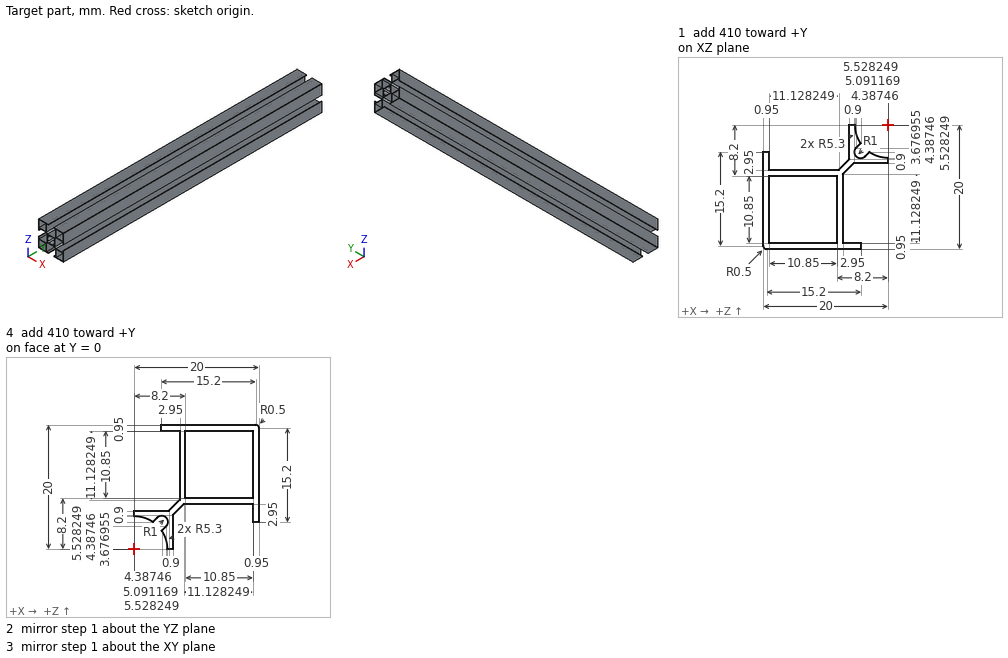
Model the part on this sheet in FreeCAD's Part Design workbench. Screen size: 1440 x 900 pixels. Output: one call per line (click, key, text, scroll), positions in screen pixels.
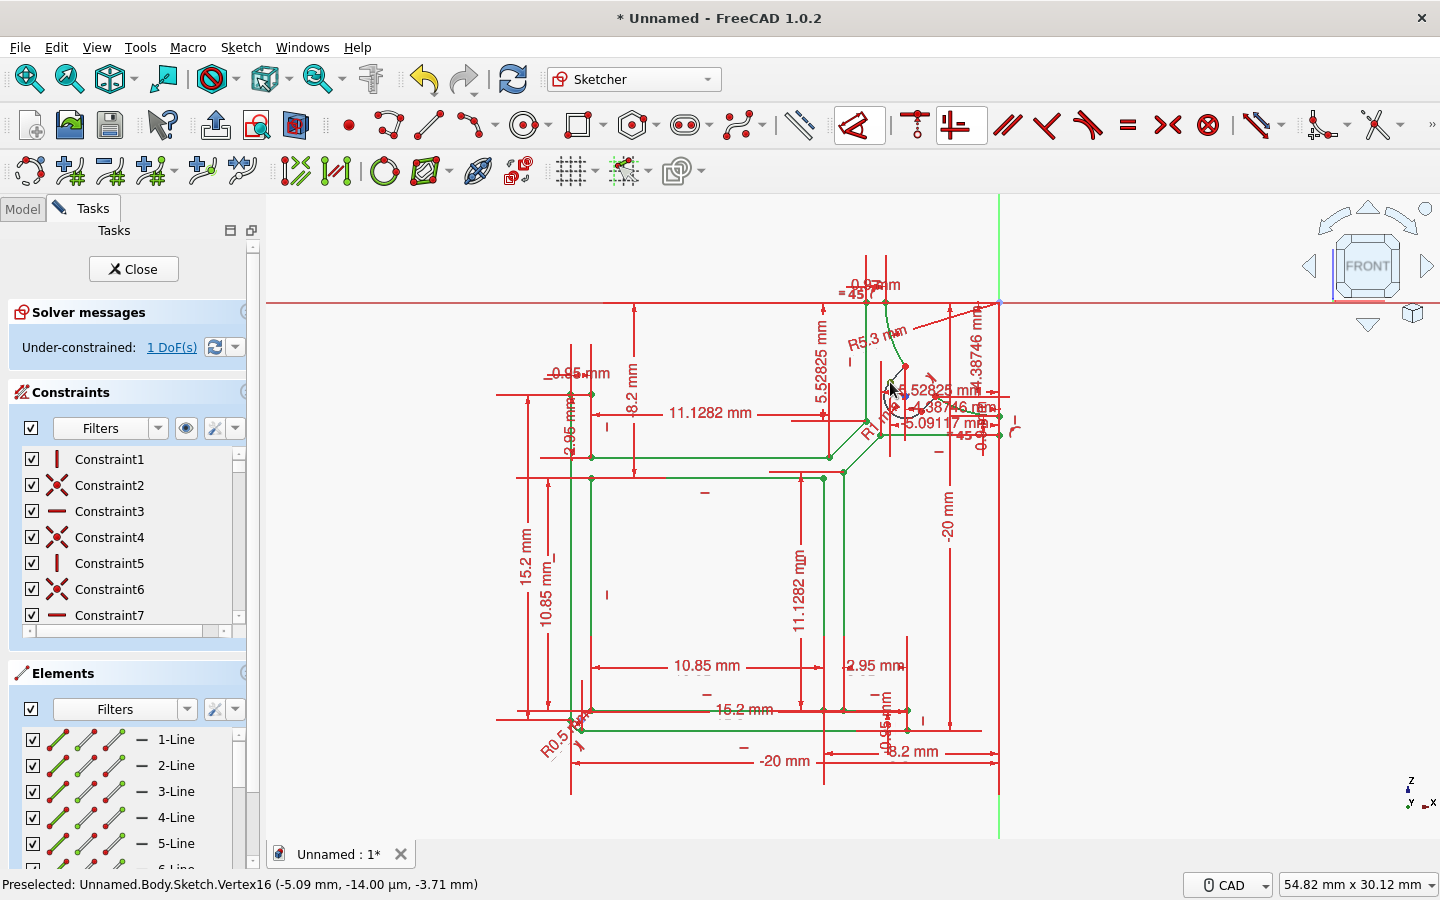
click(880, 126)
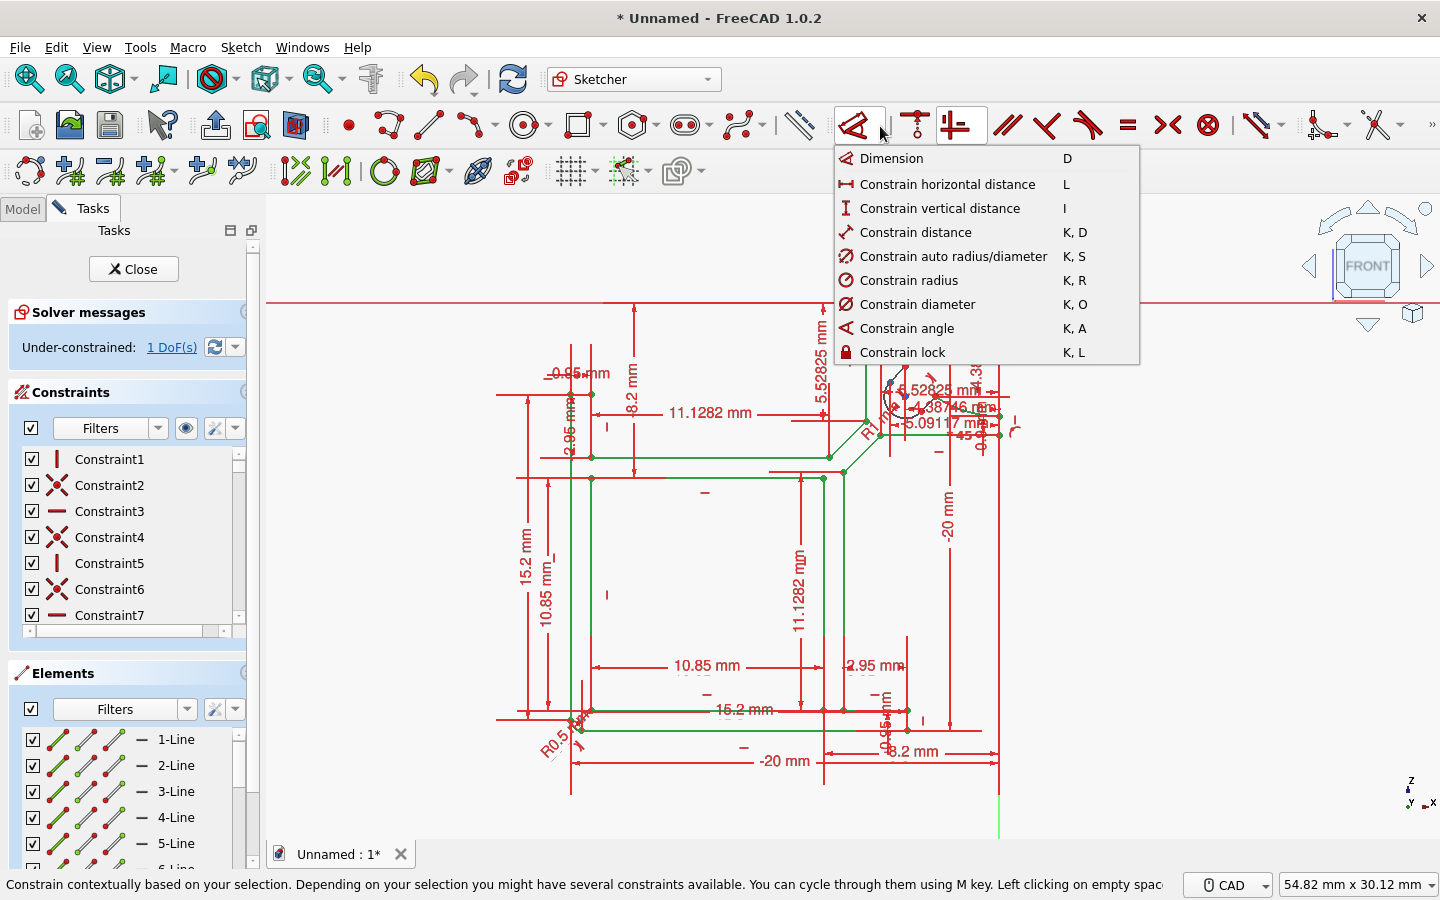
click(987, 208)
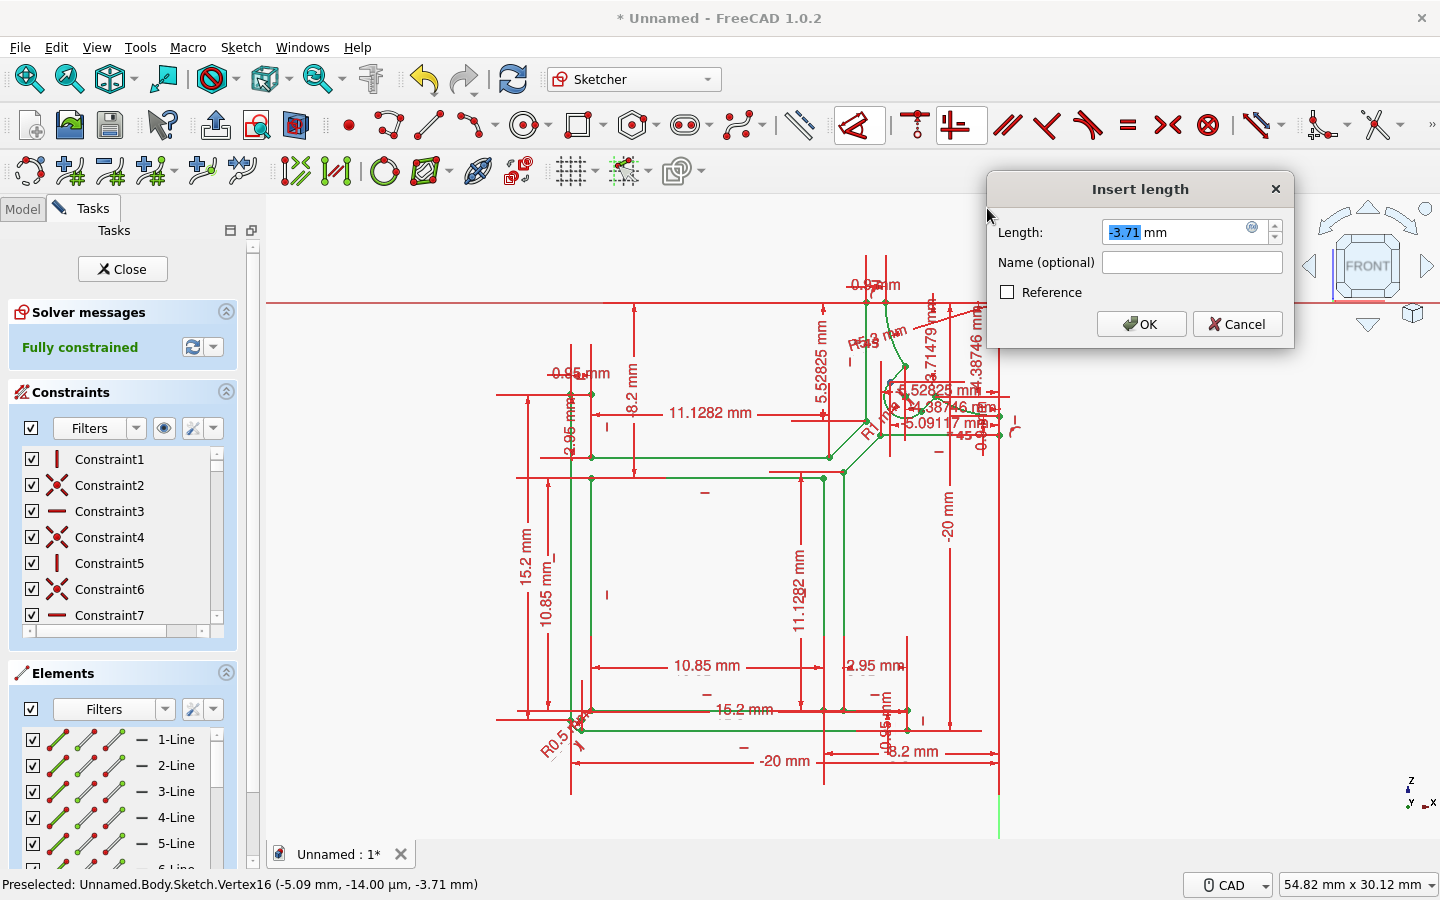
text(-3.676955)
key(Return)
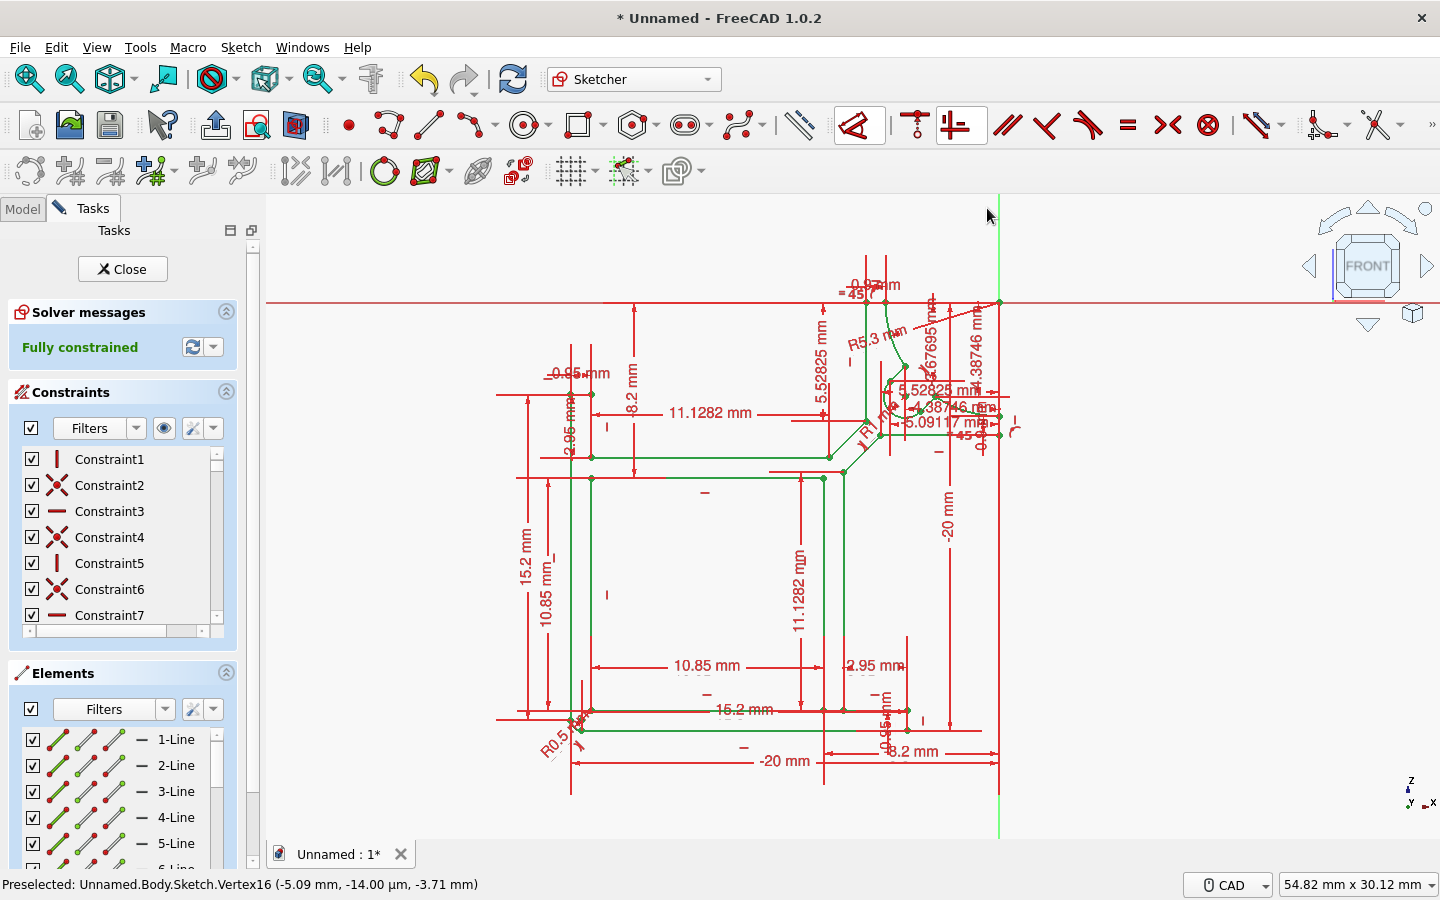
click(123, 269)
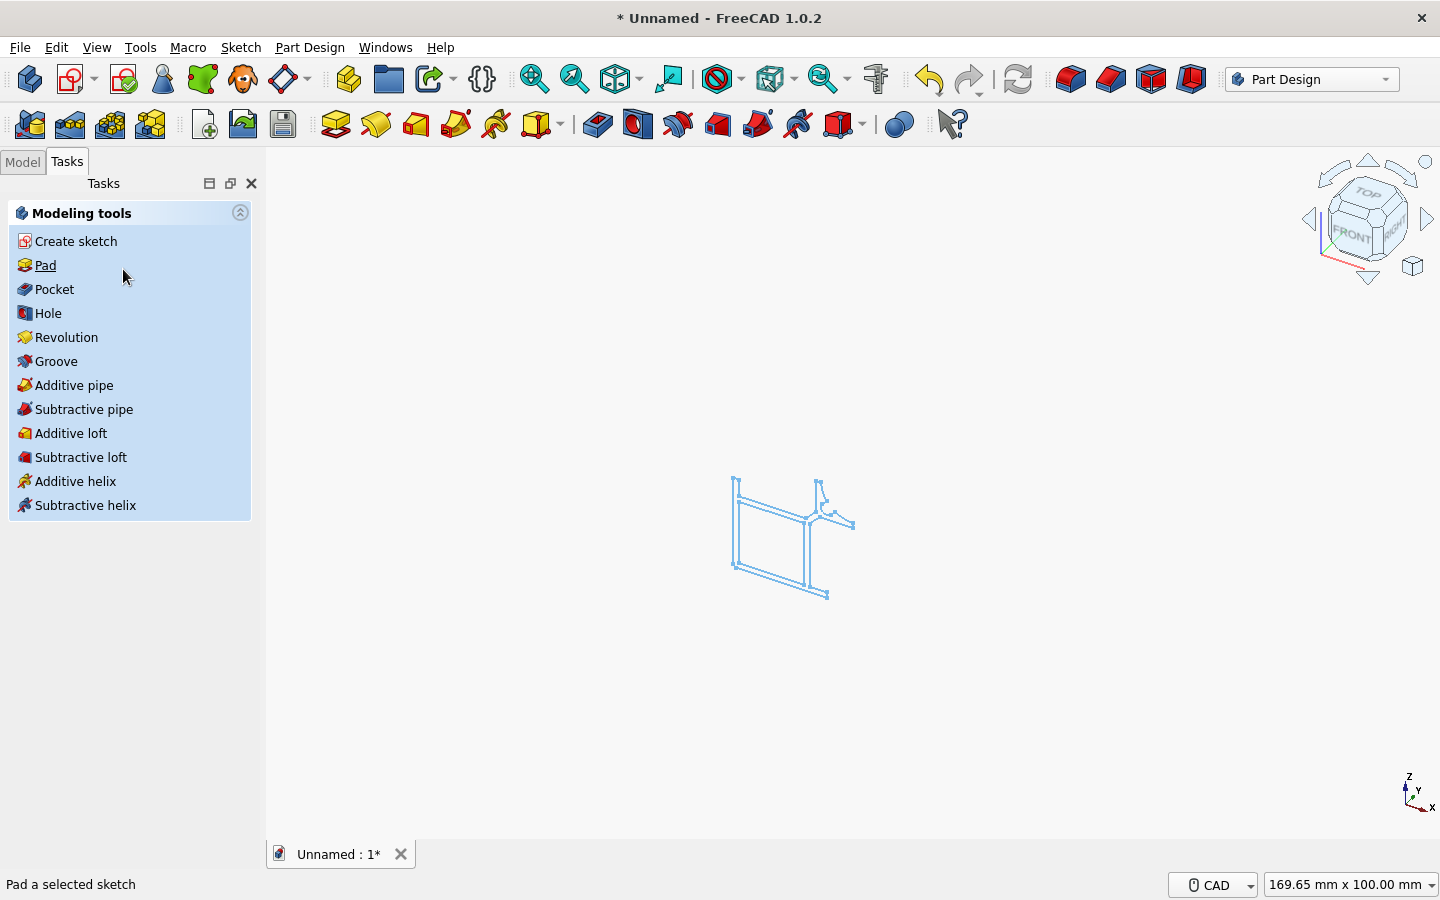
click(336, 124)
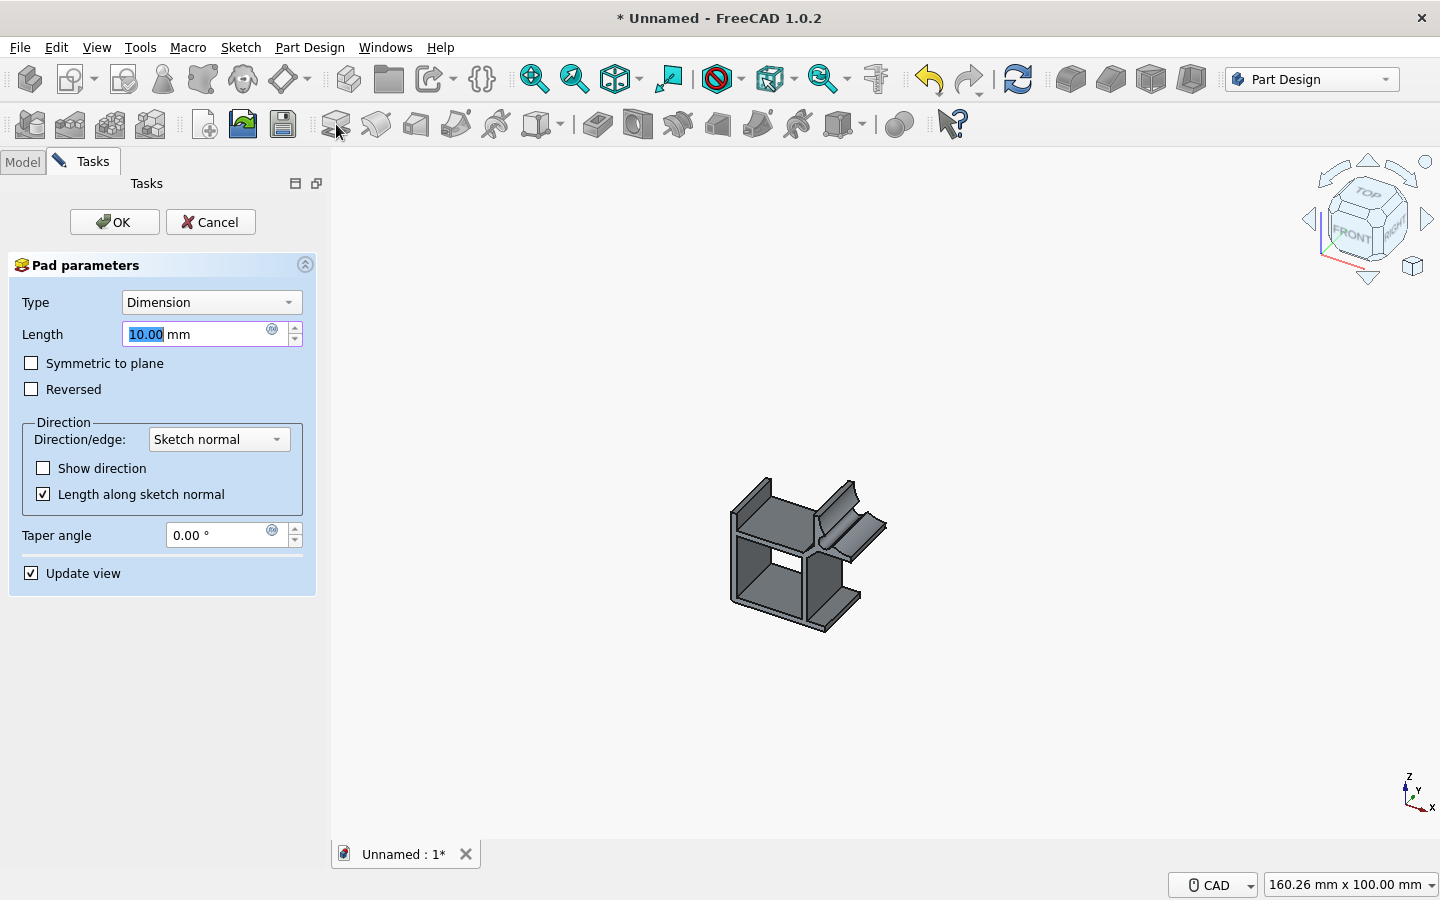
text(410)
key(Tab)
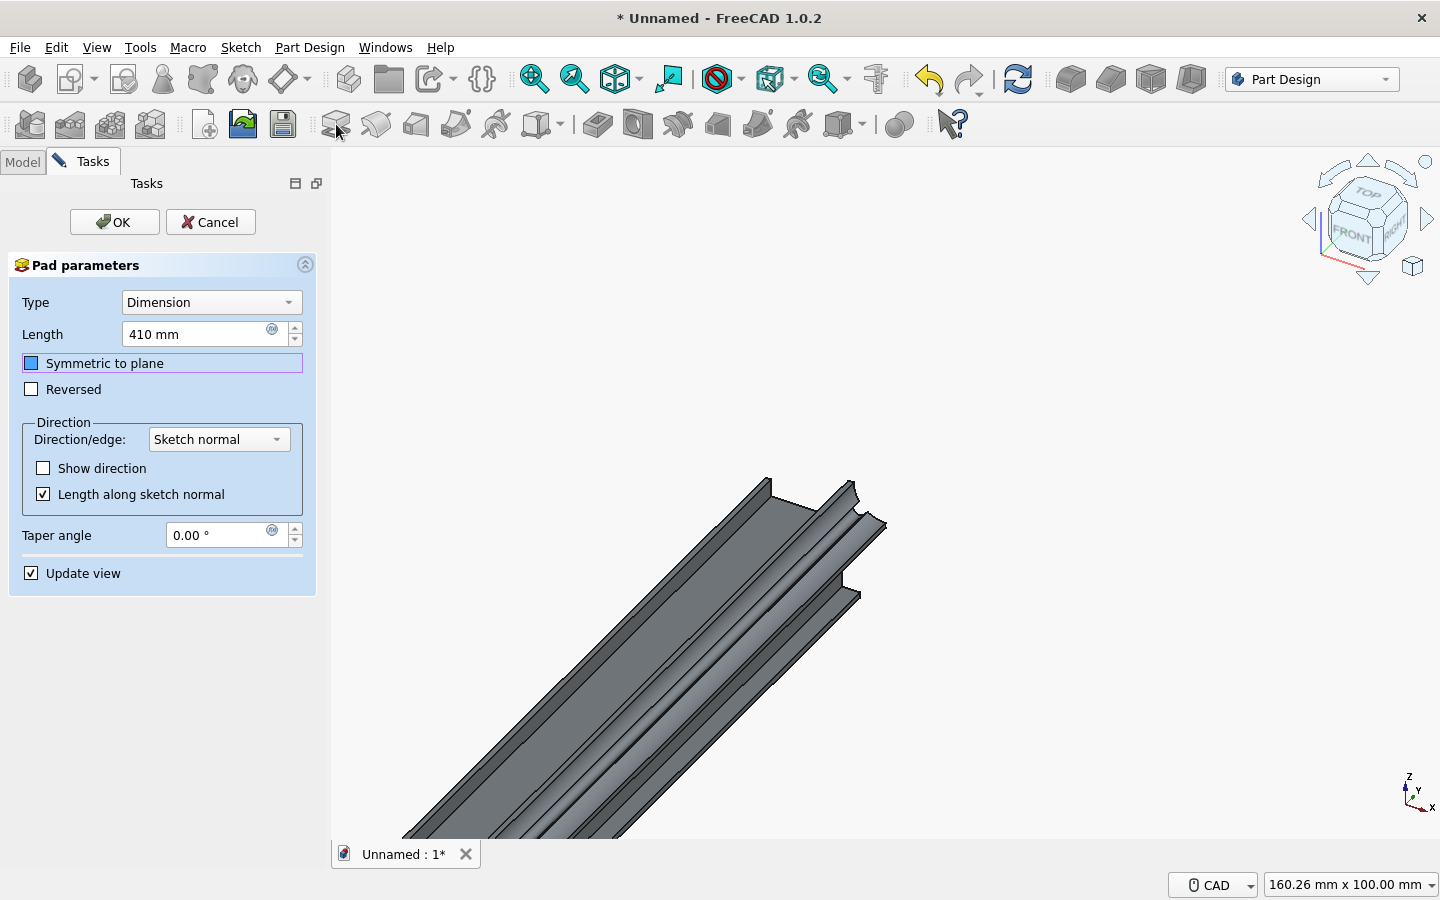
click(30, 389)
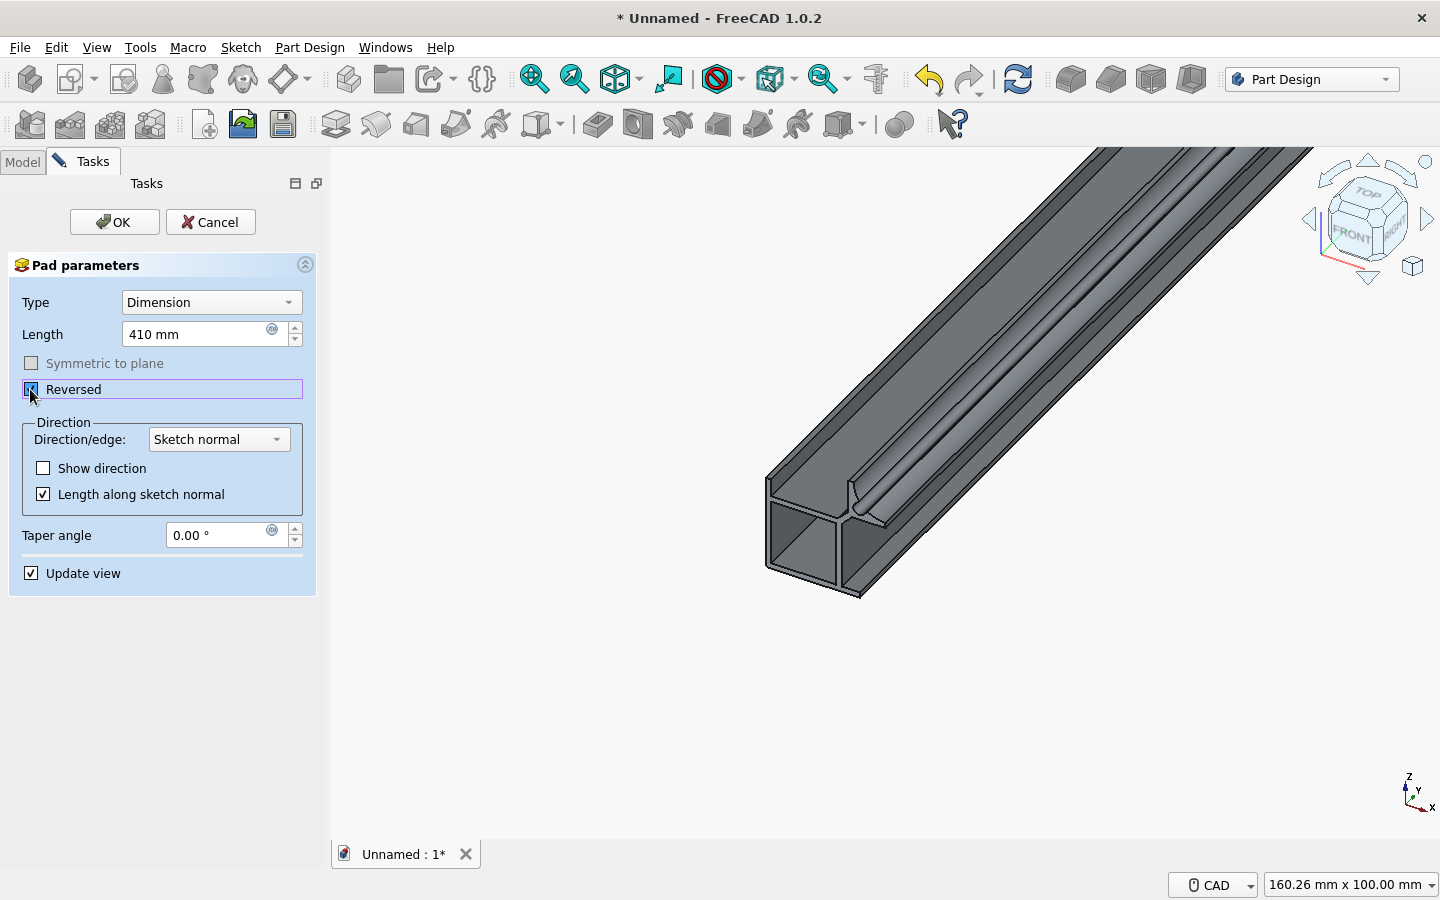
click(115, 222)